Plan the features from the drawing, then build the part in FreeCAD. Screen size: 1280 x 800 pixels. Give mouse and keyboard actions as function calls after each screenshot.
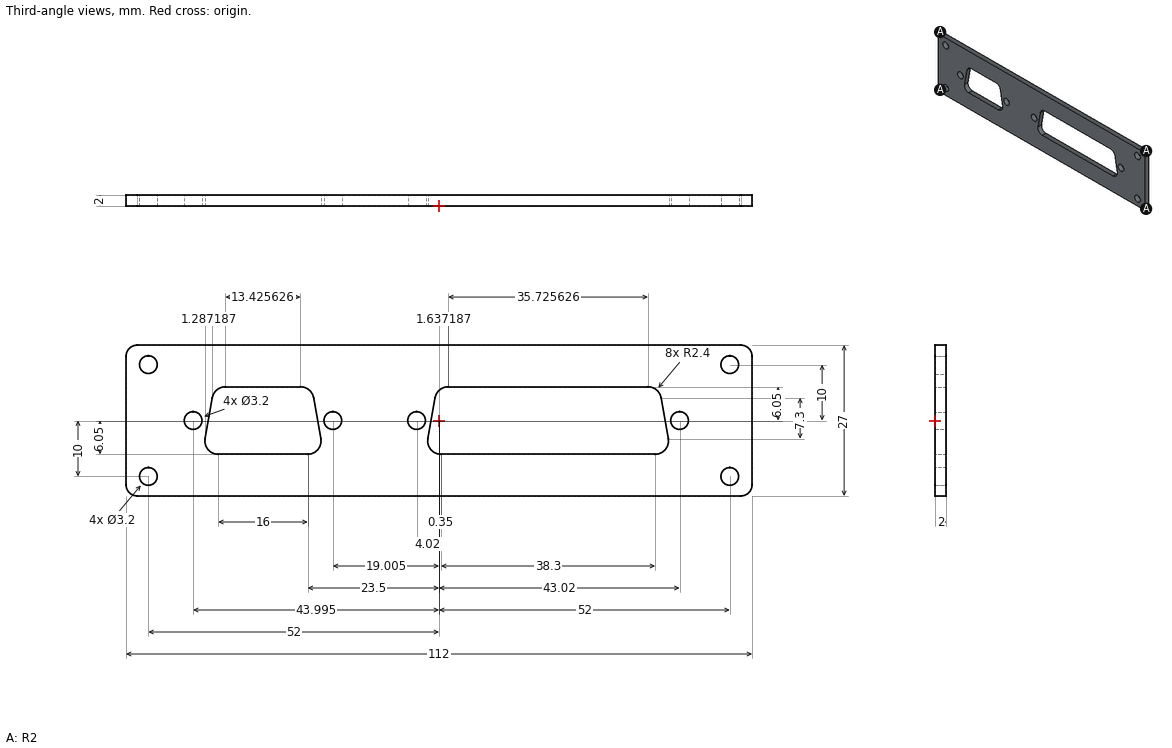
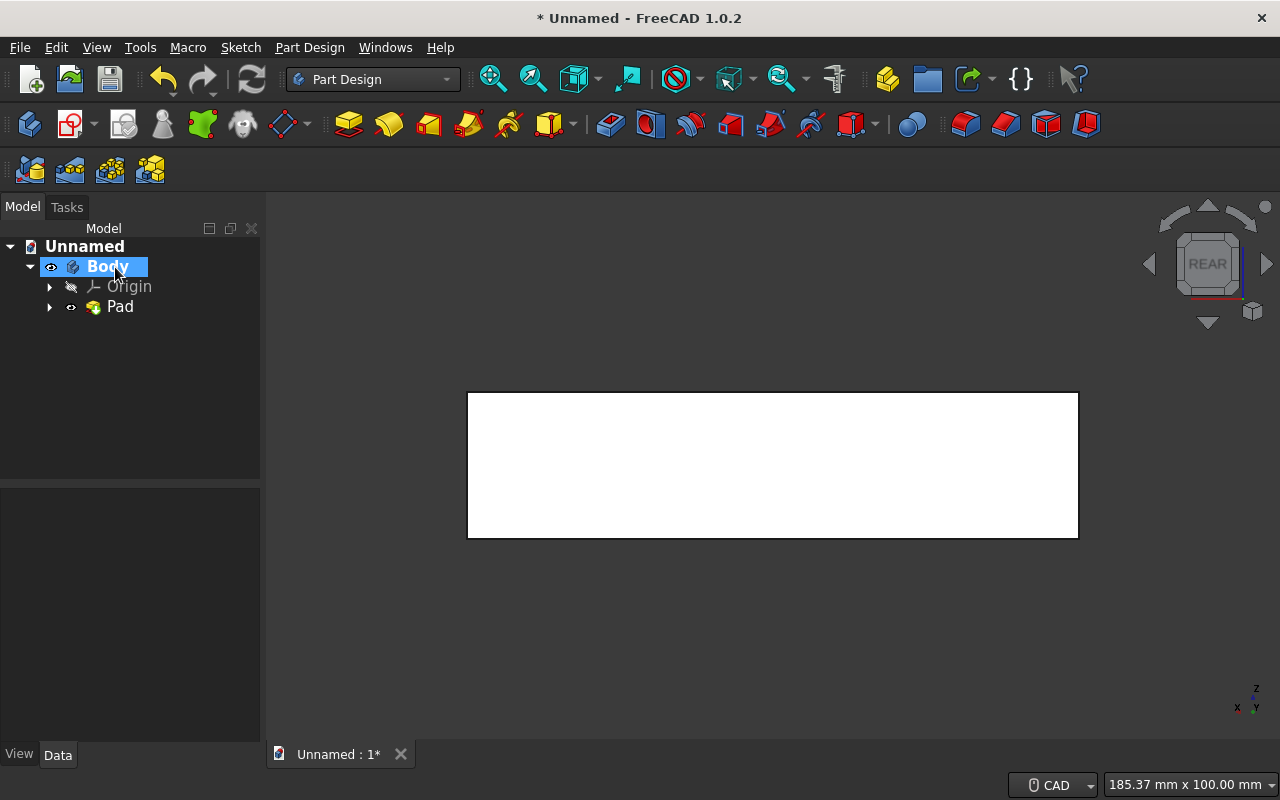
click(598, 464)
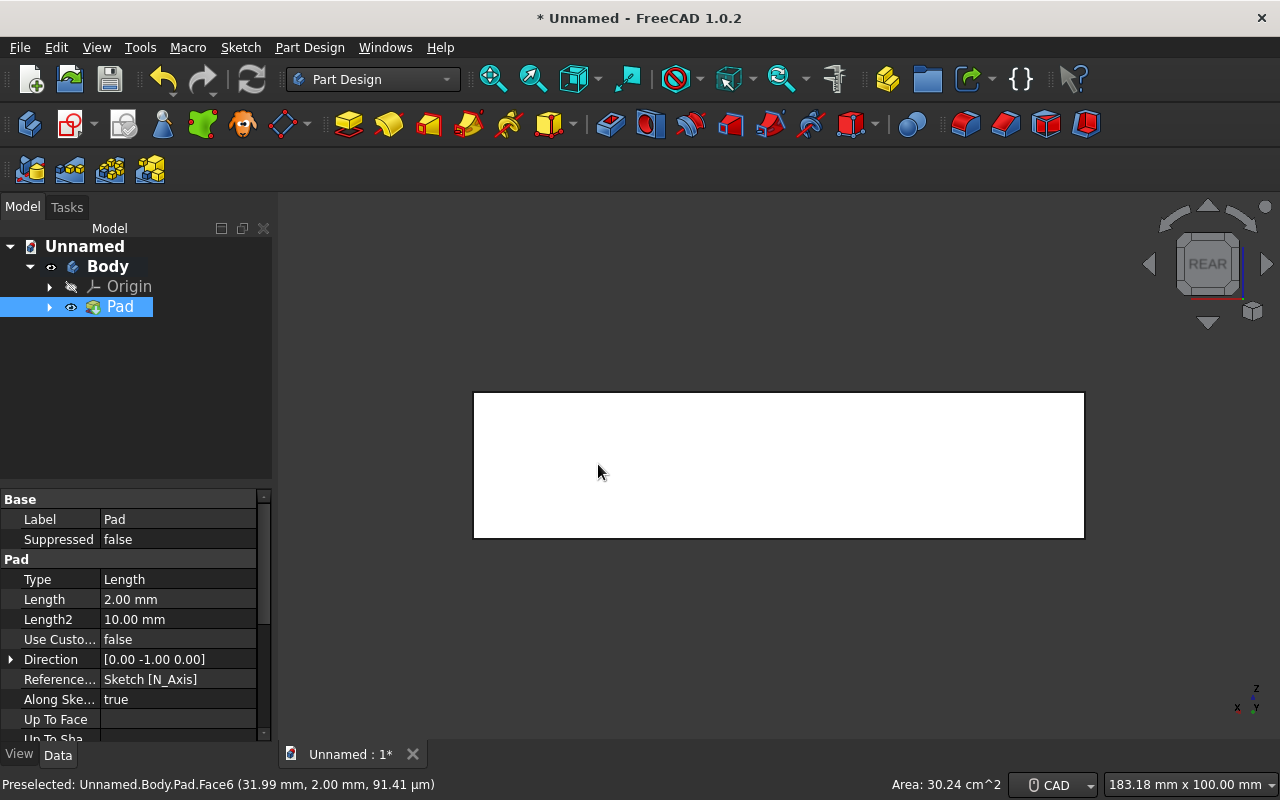
click(70, 124)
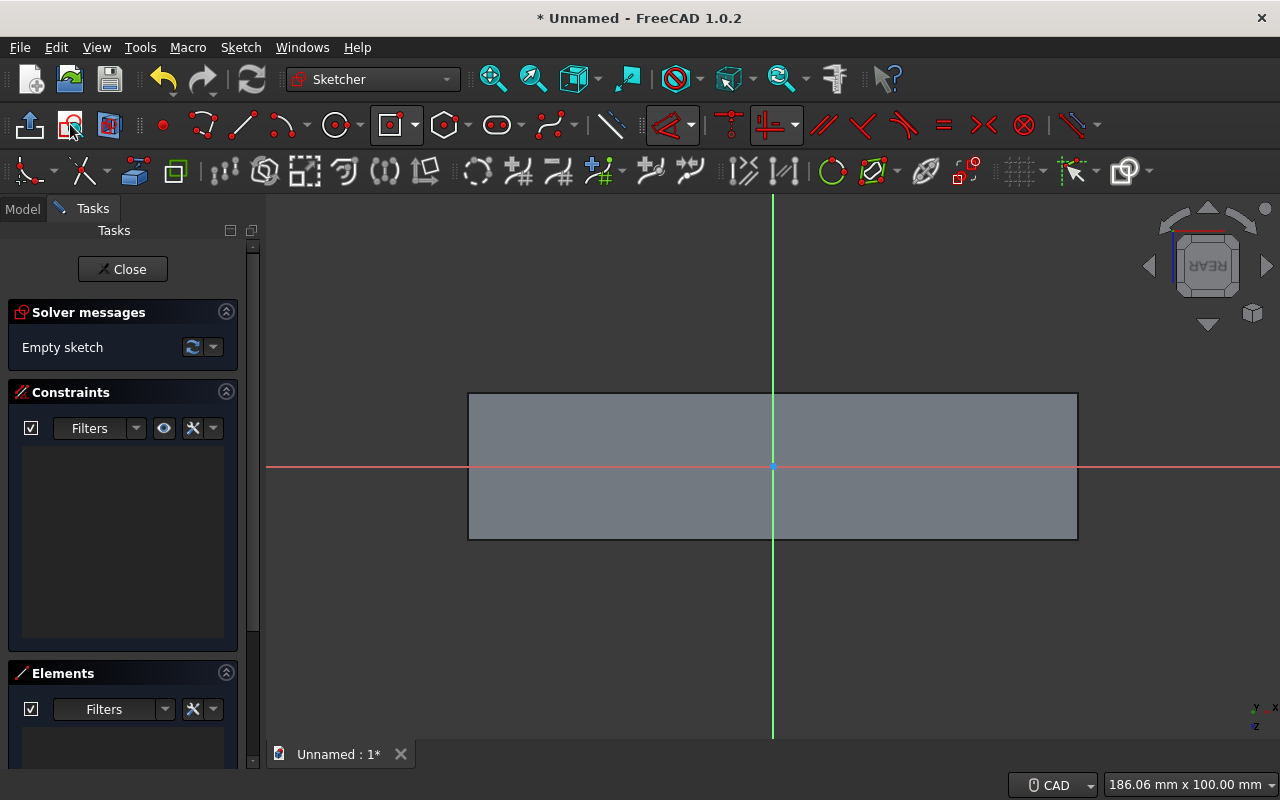
click(336, 126)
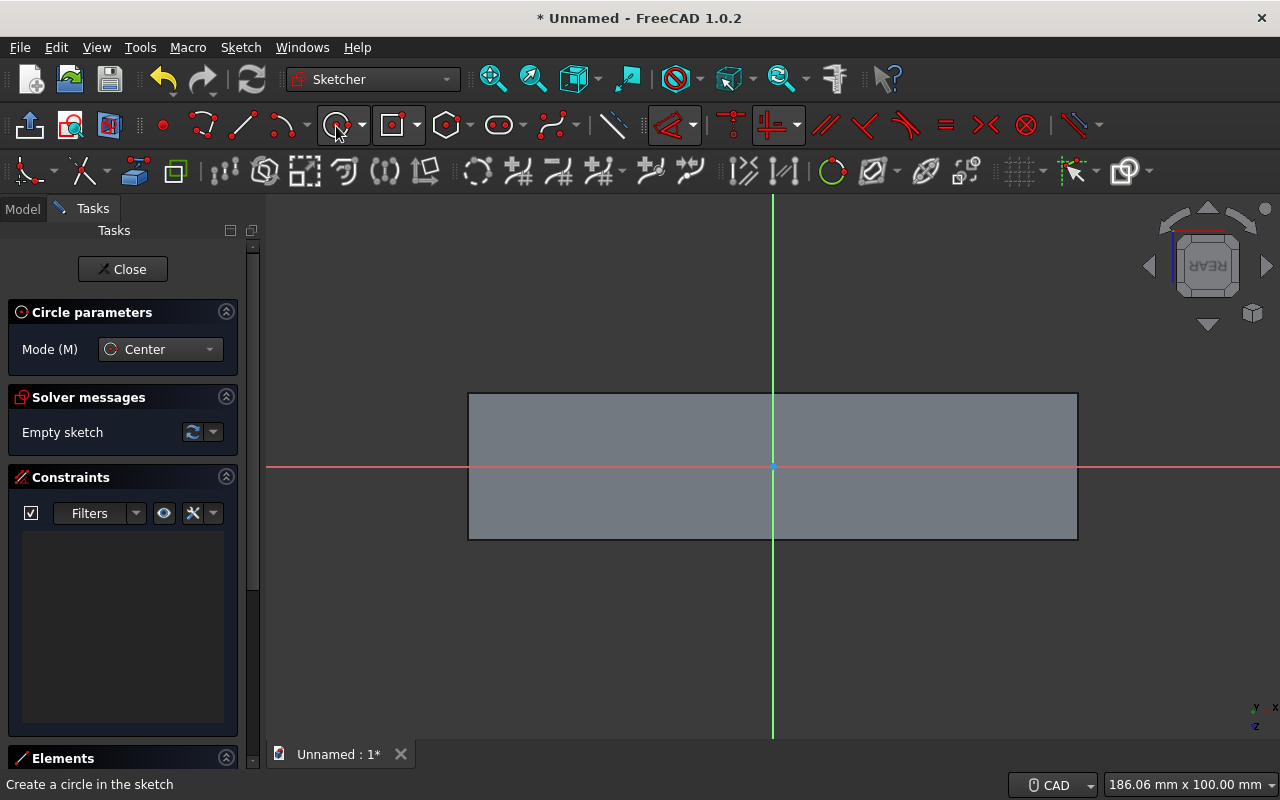
scroll(490, 412, up, 5)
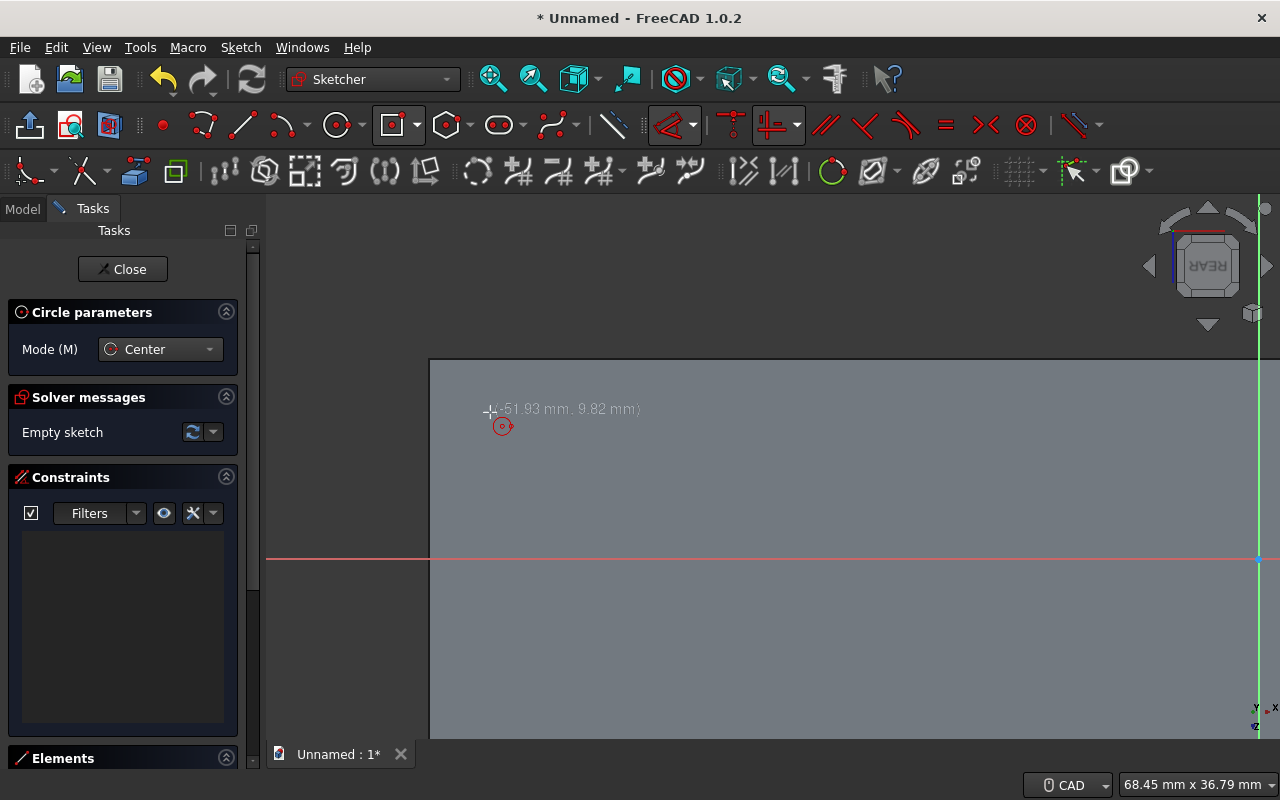
click(489, 411)
click(505, 395)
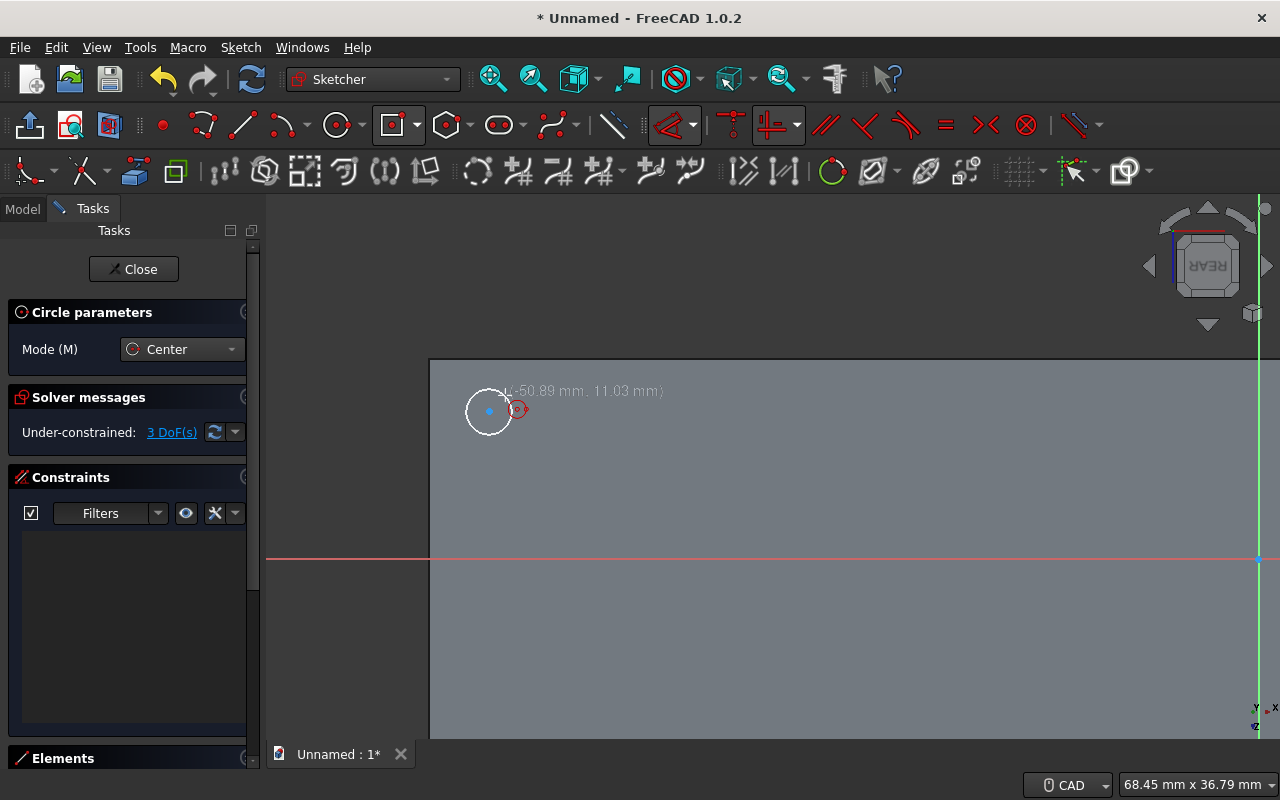
scroll(382, 412, down, 5)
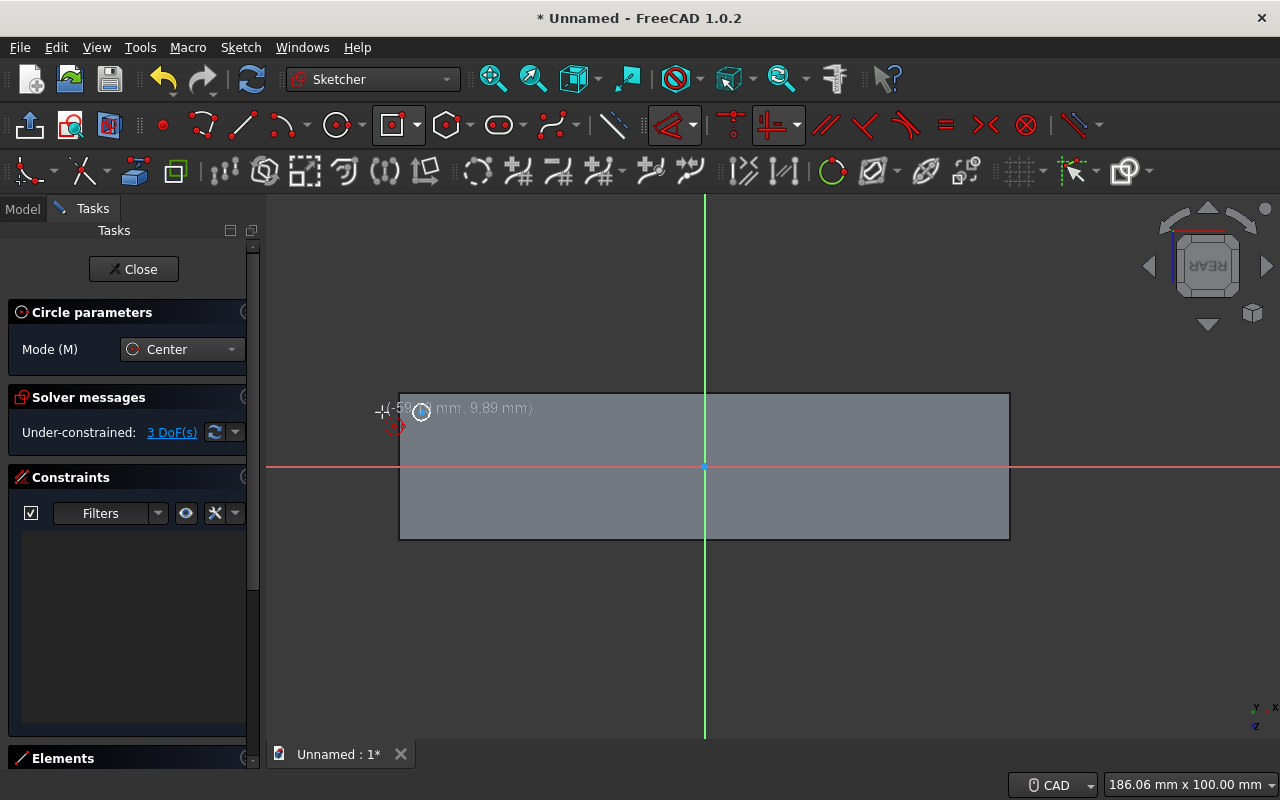
scroll(988, 412, up, 5)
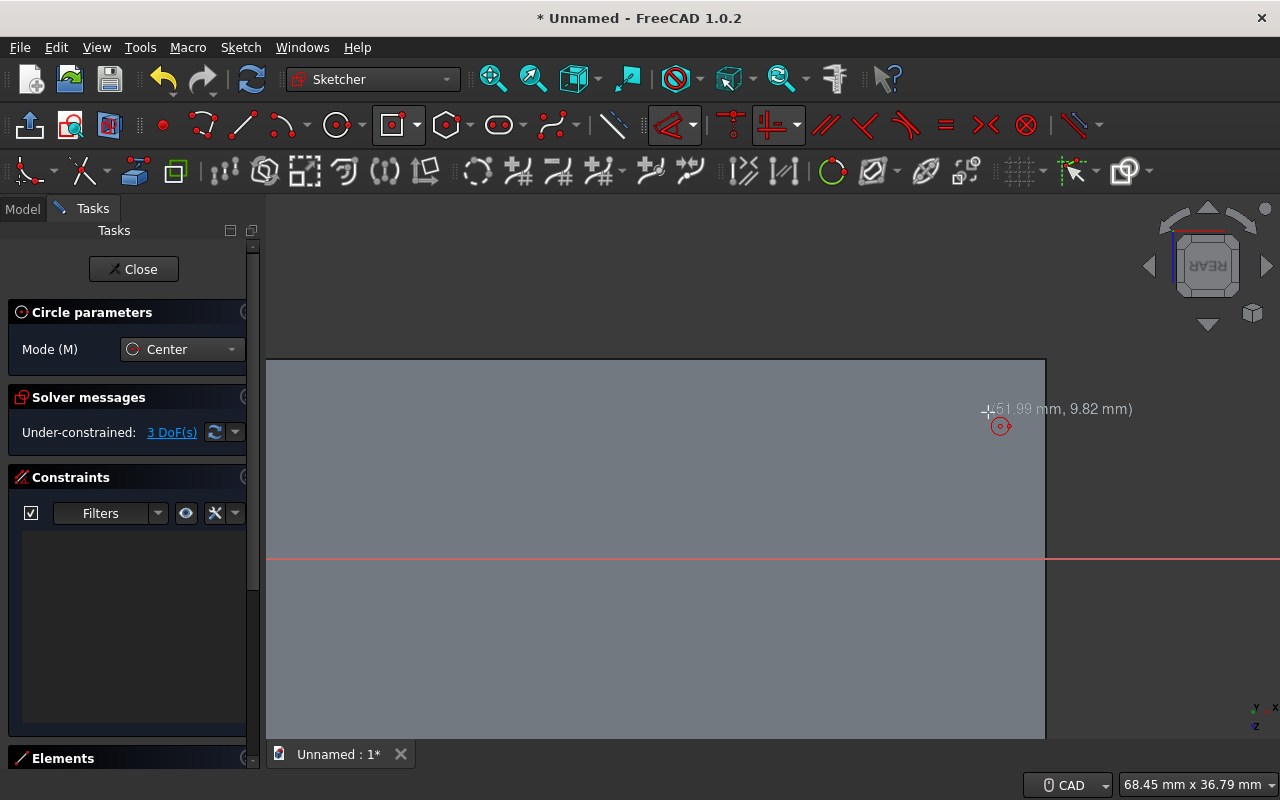
click(987, 411)
click(1004, 395)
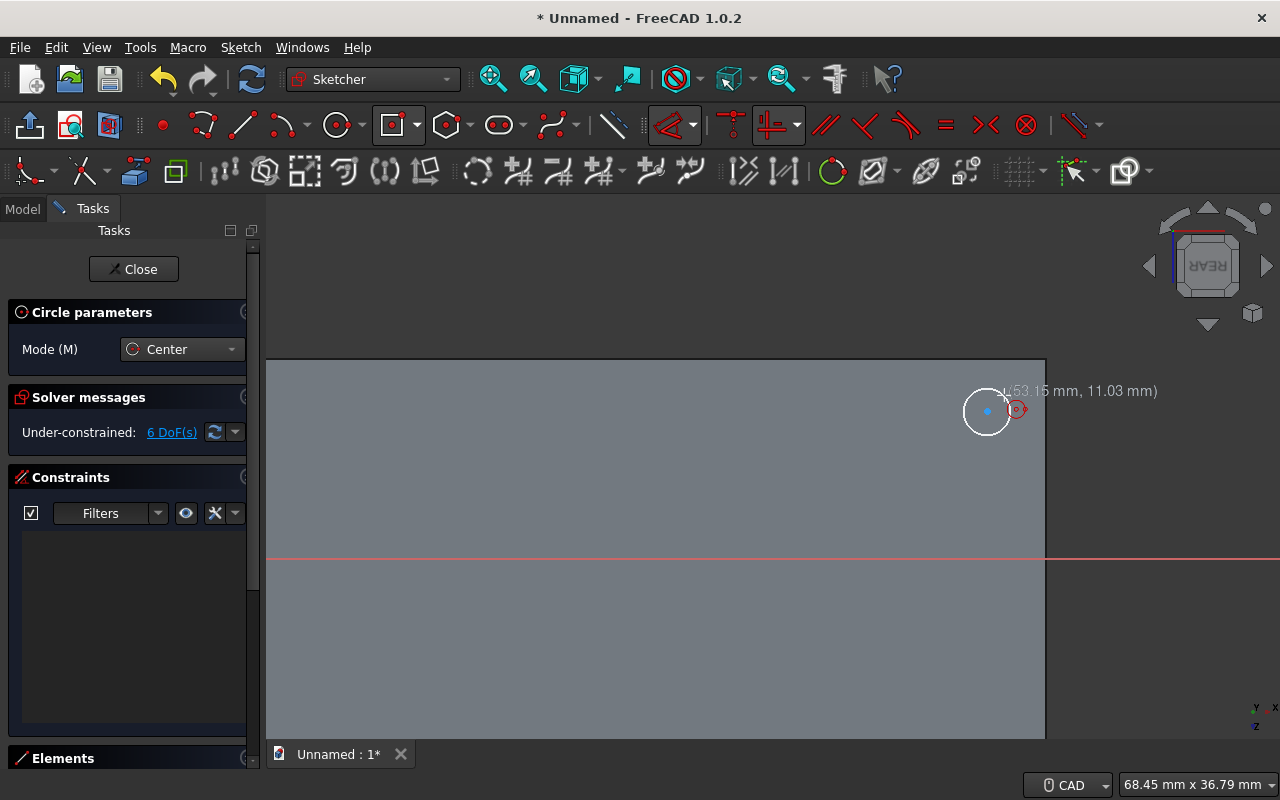
click(987, 708)
click(1004, 691)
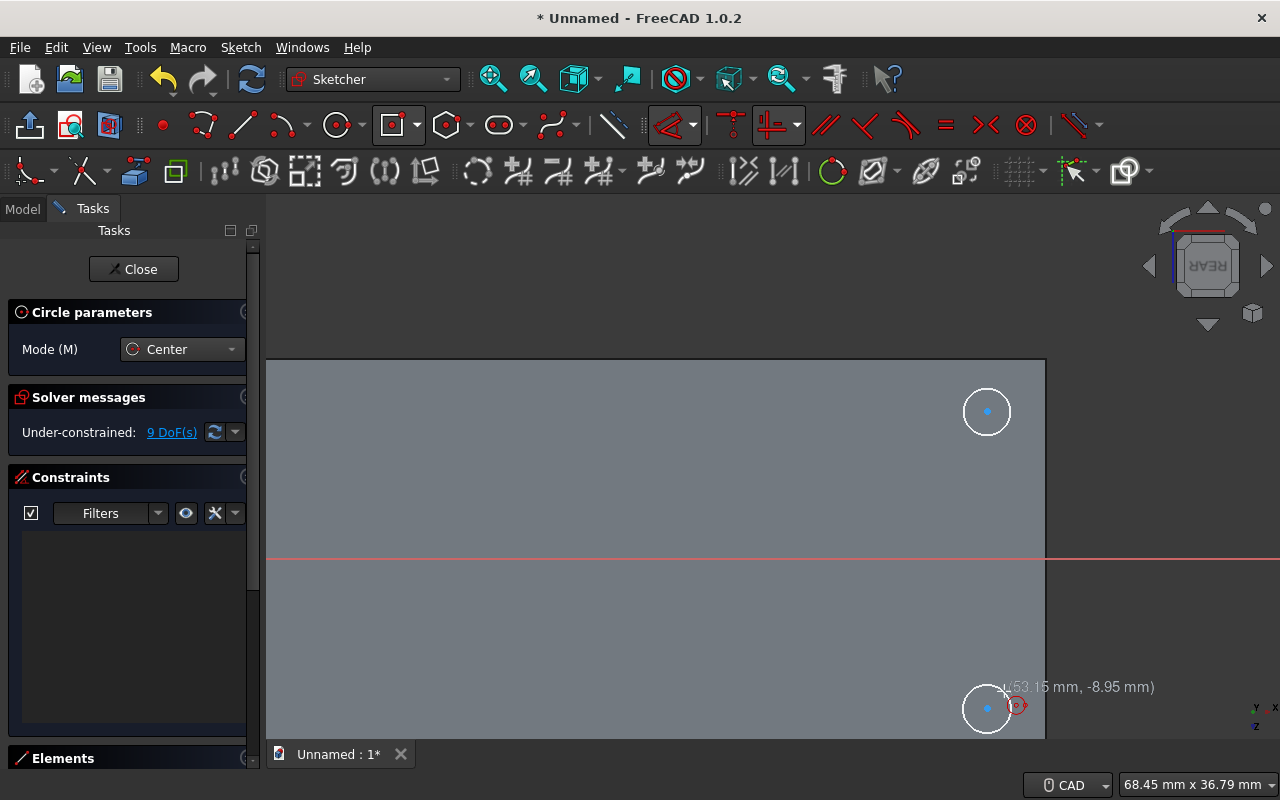
scroll(988, 412, down, 5)